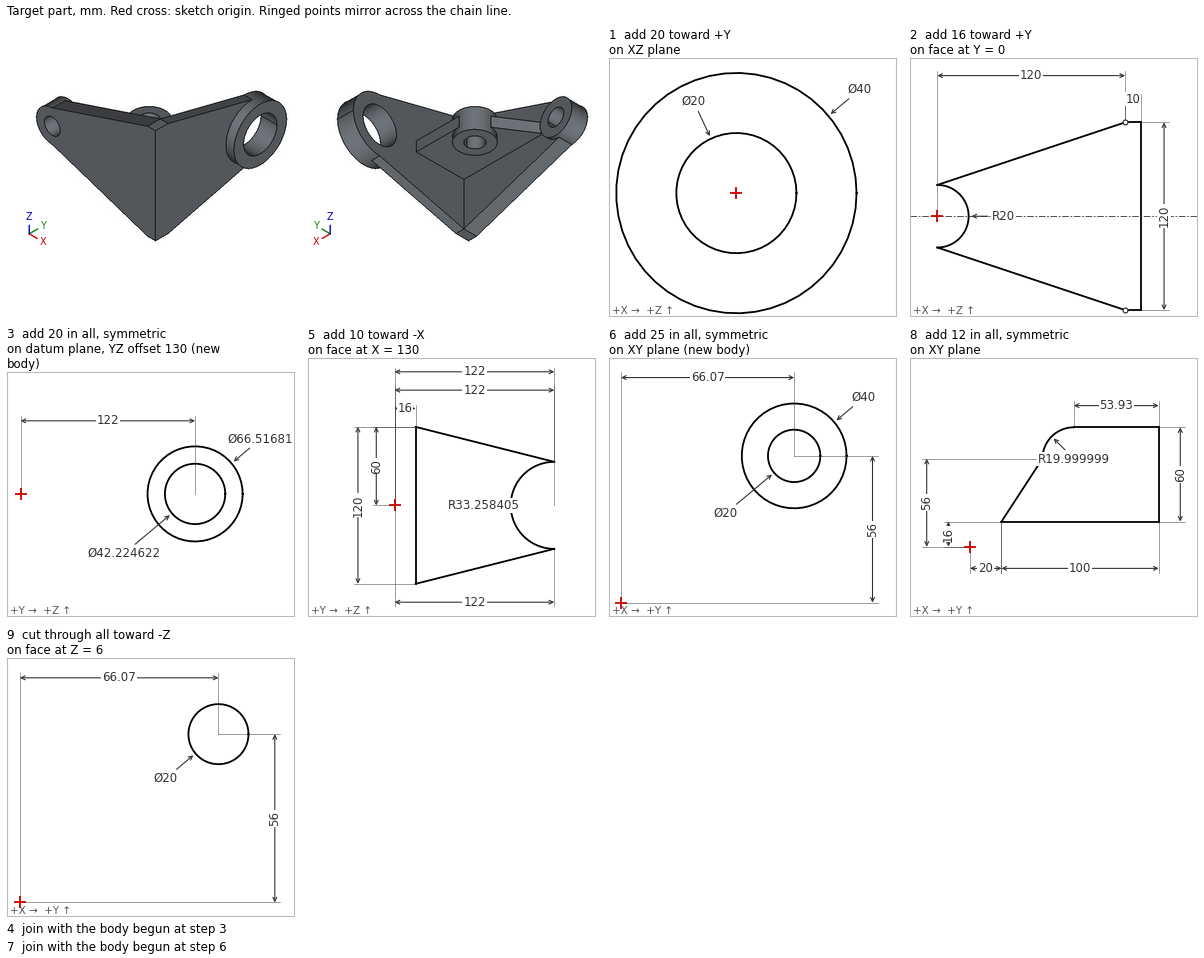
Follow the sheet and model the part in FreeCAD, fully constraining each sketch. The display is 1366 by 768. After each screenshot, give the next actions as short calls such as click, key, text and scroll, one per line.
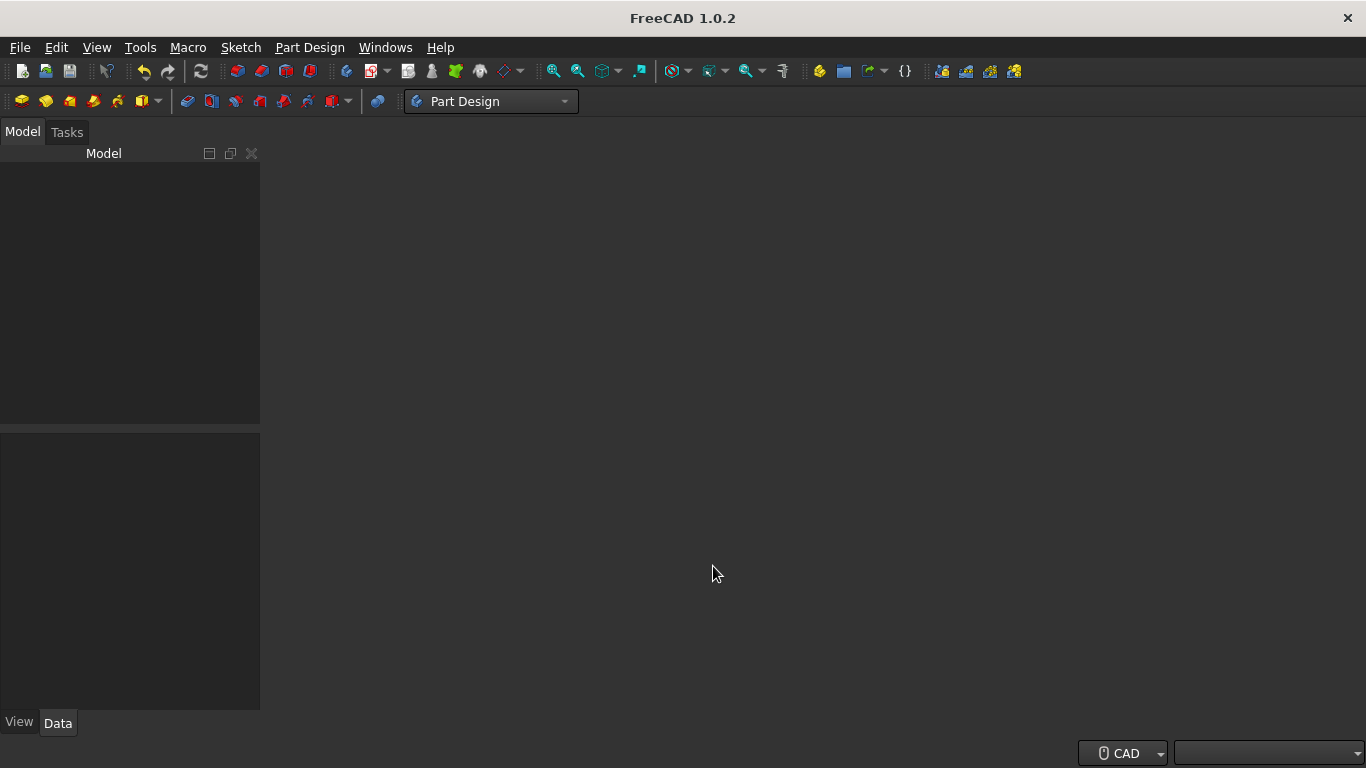
click(22, 72)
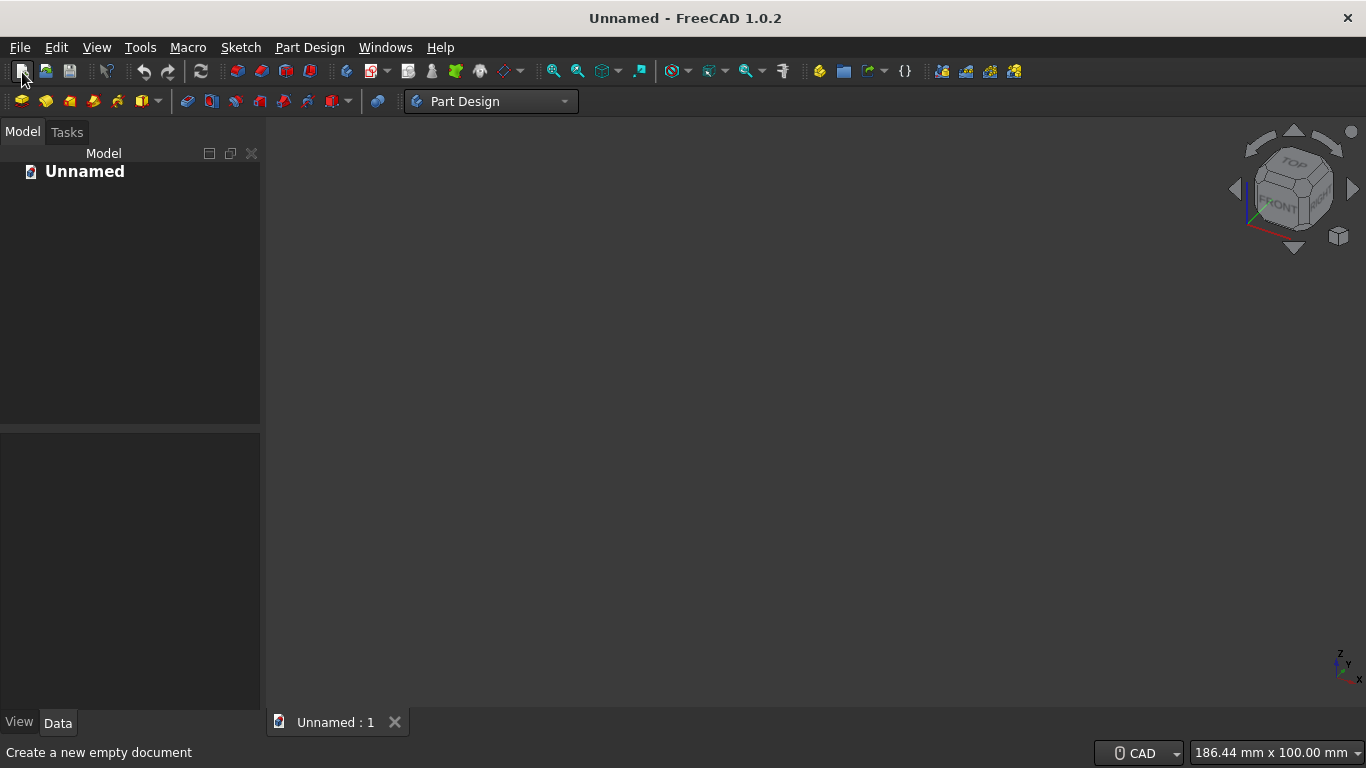
click(372, 72)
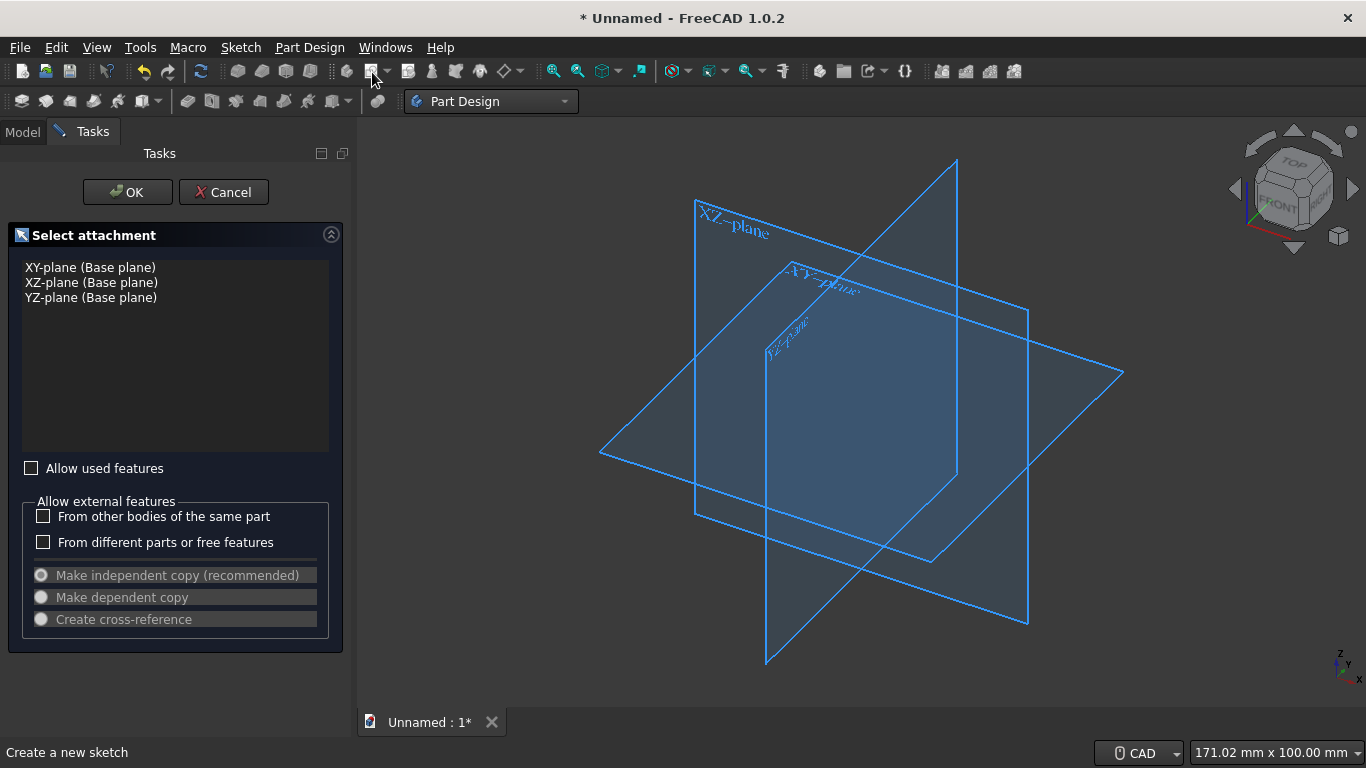
click(82, 282)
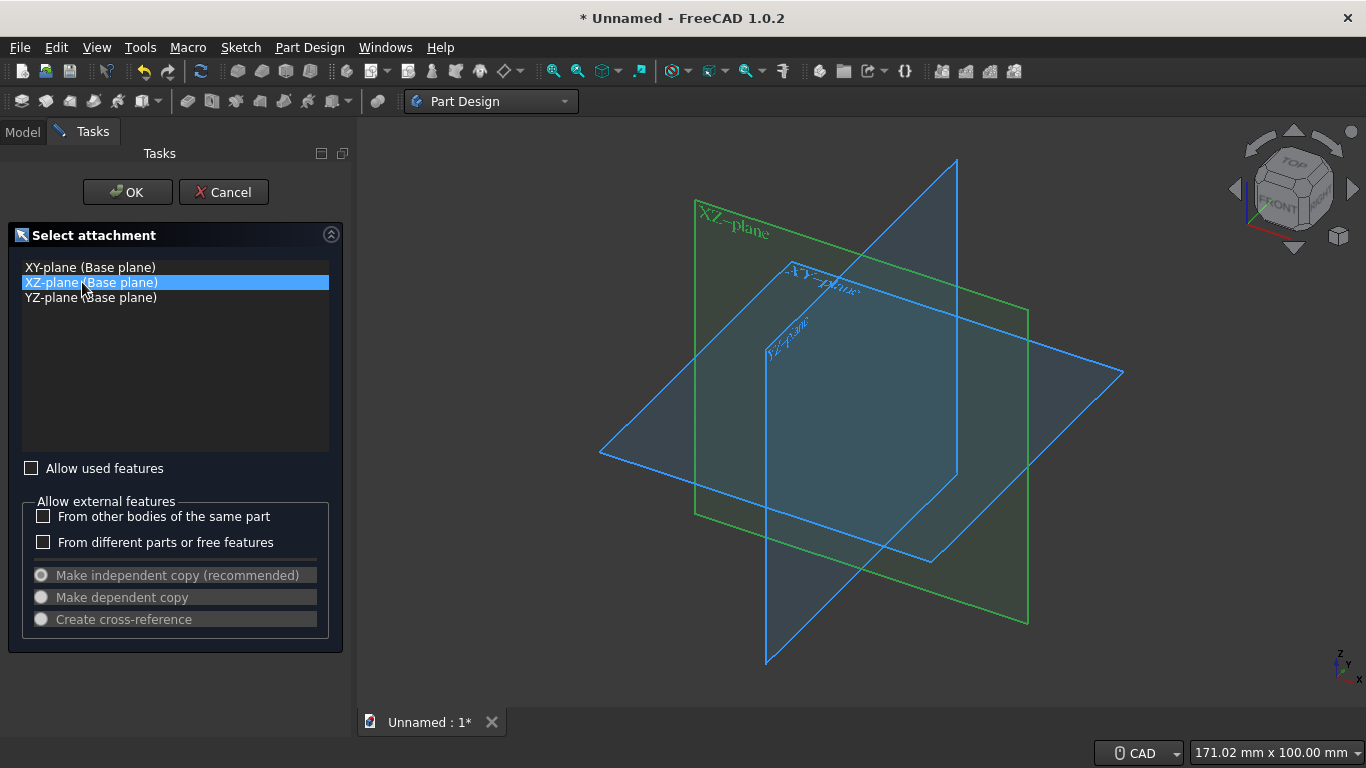
click(128, 192)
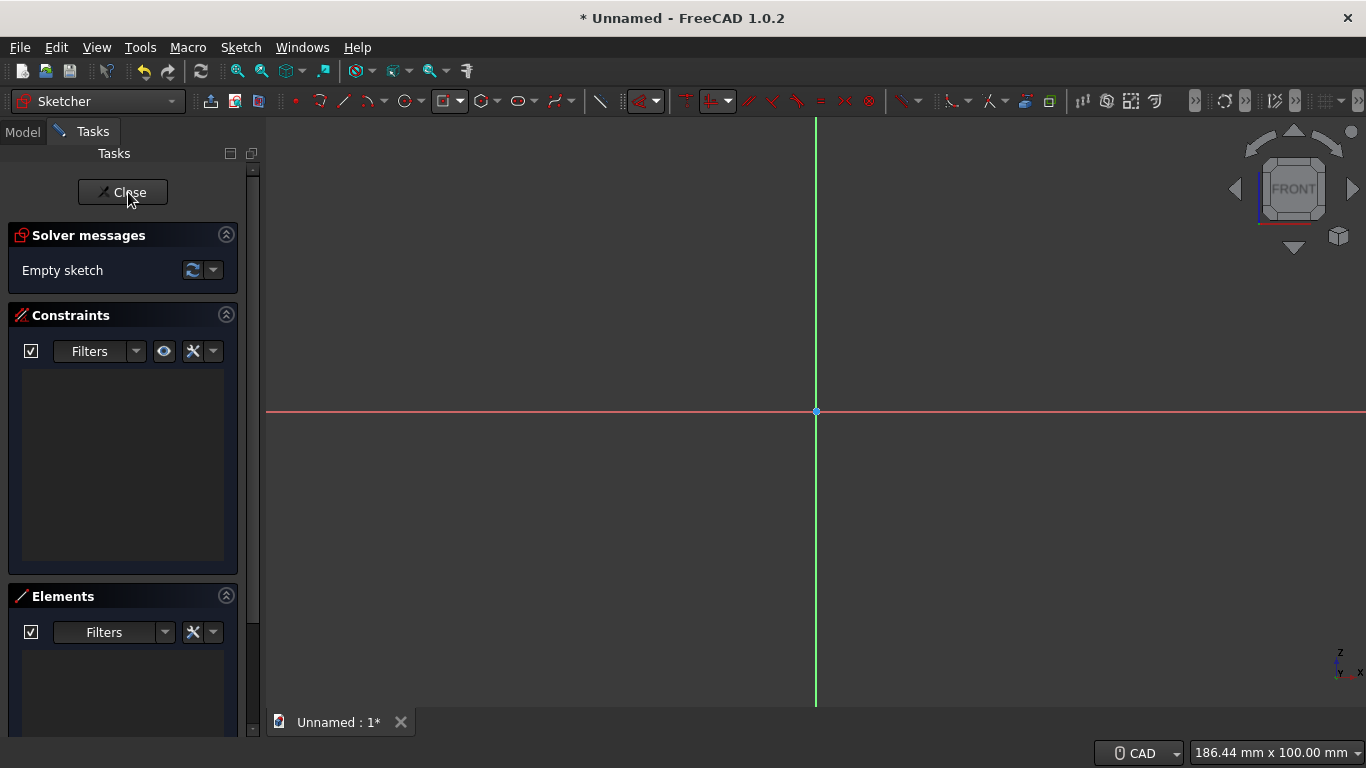
scroll(955, 412, up, 2)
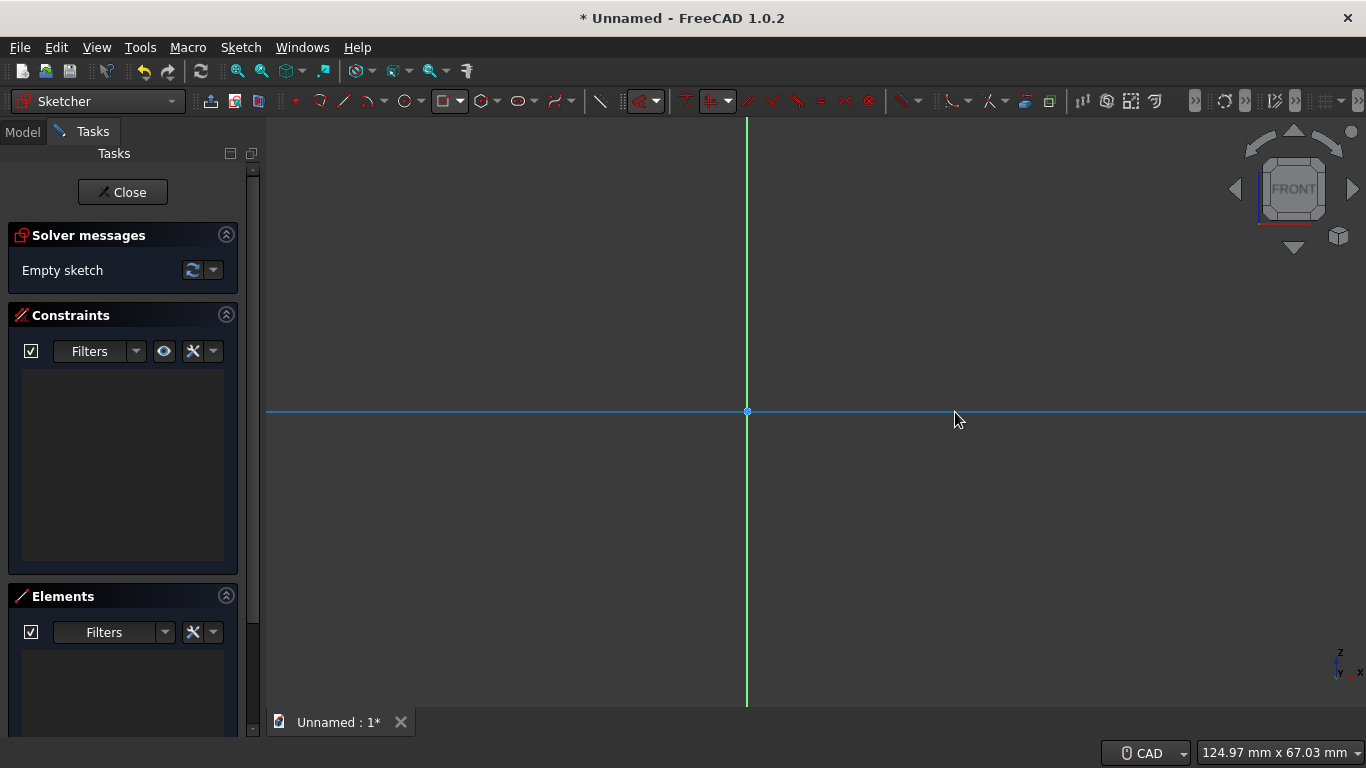
key(g)
key(c)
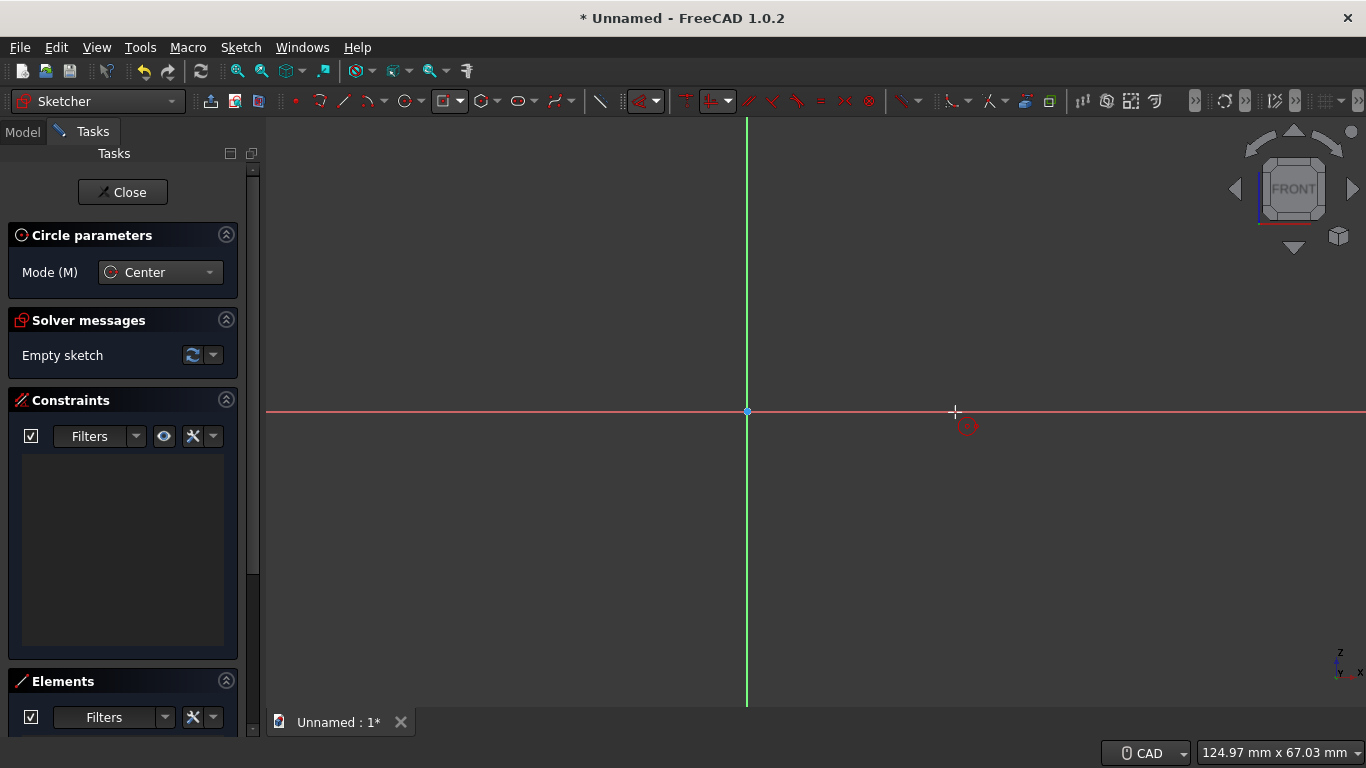
click(747, 412)
click(872, 287)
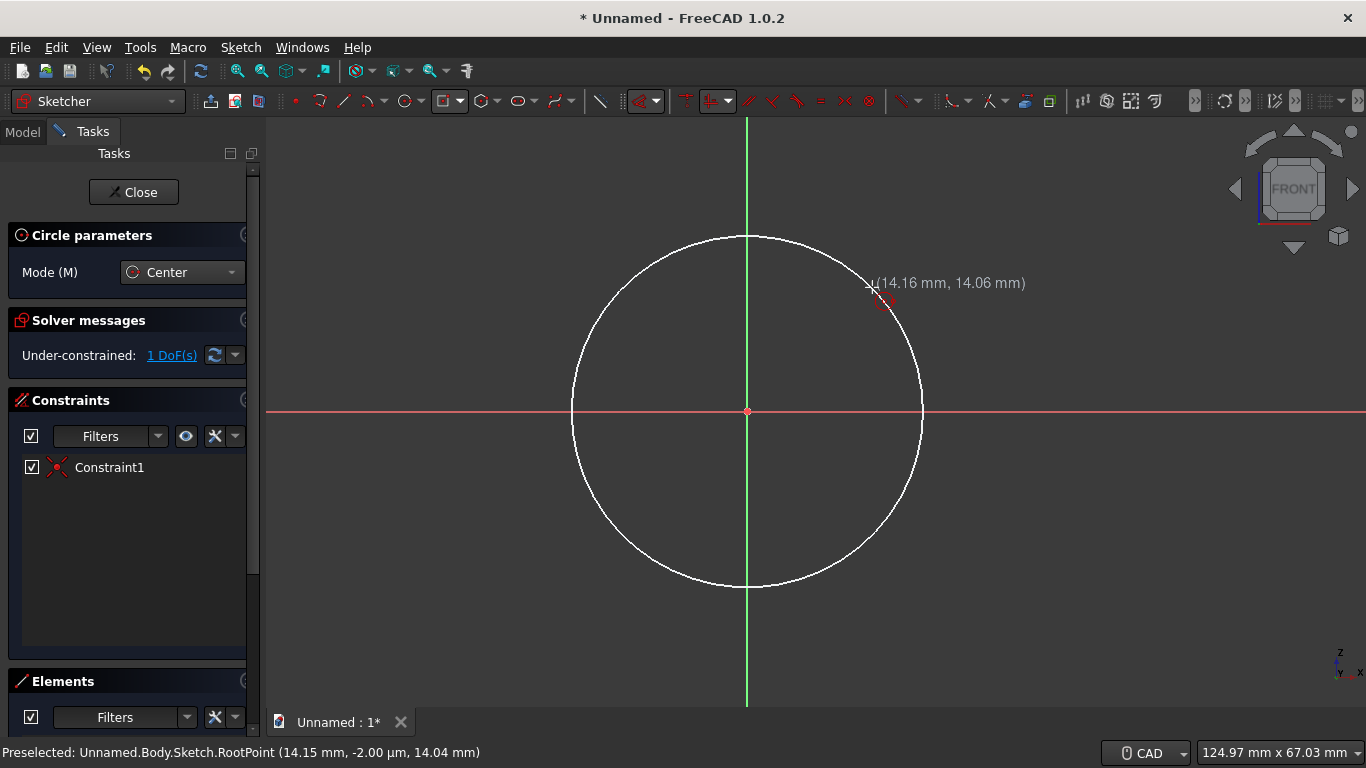
click(747, 412)
click(810, 350)
key(Escape)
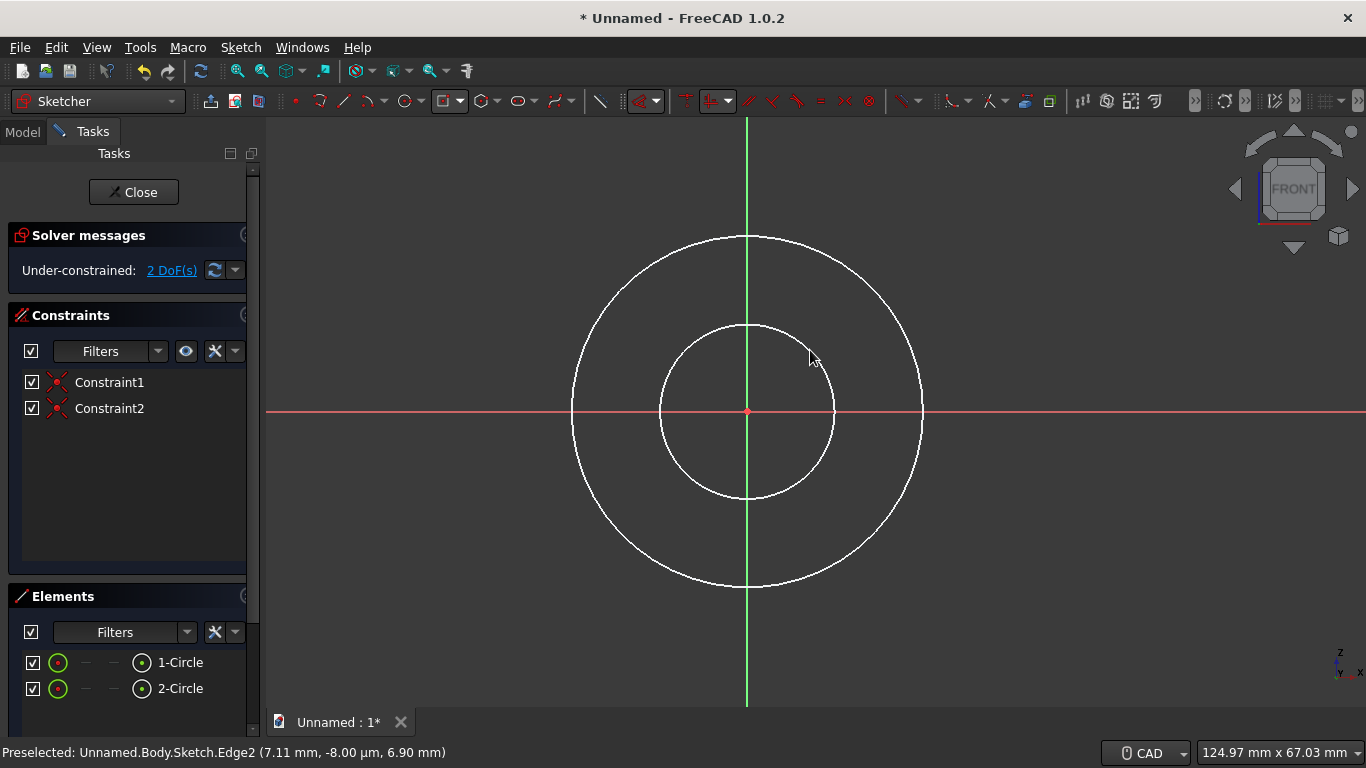
click(640, 102)